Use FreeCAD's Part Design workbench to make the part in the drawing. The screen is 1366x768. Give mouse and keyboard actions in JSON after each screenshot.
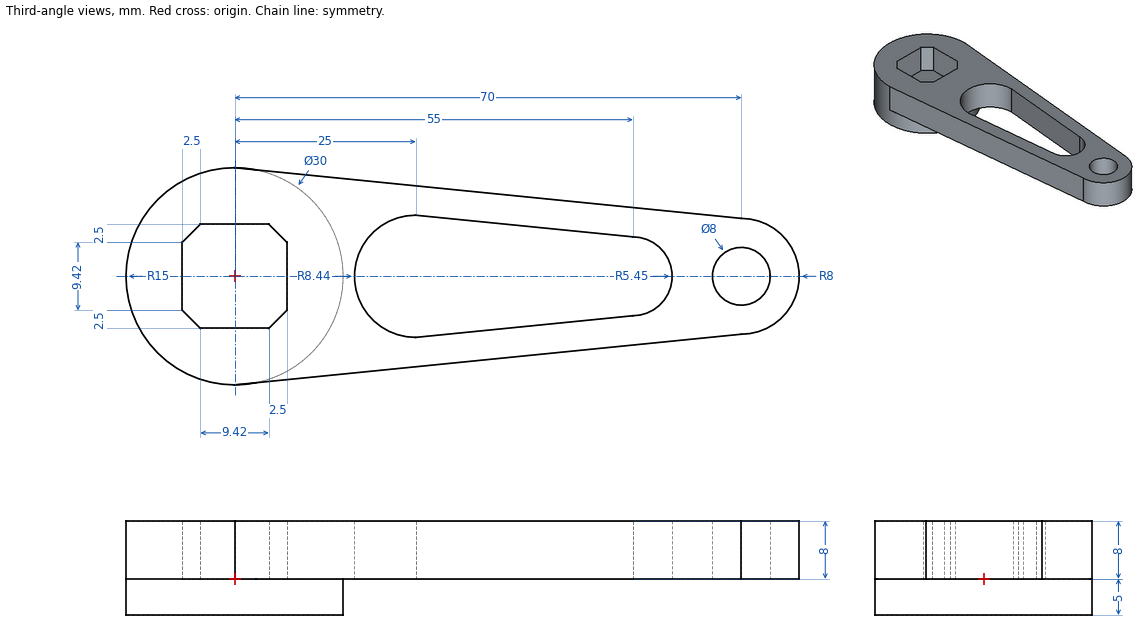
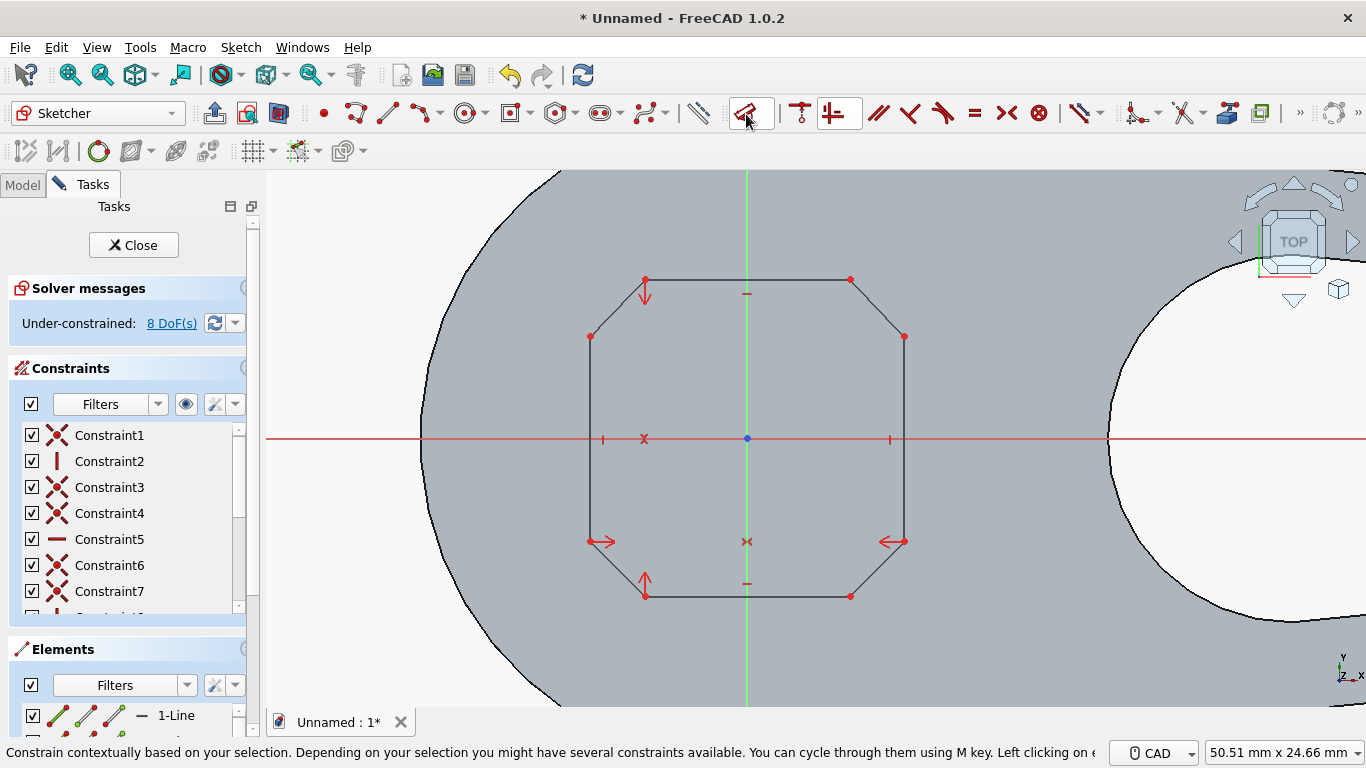
{"action": "left_click", "coordinate": [590, 398]}
{"action": "left_click", "coordinate": [556, 392]}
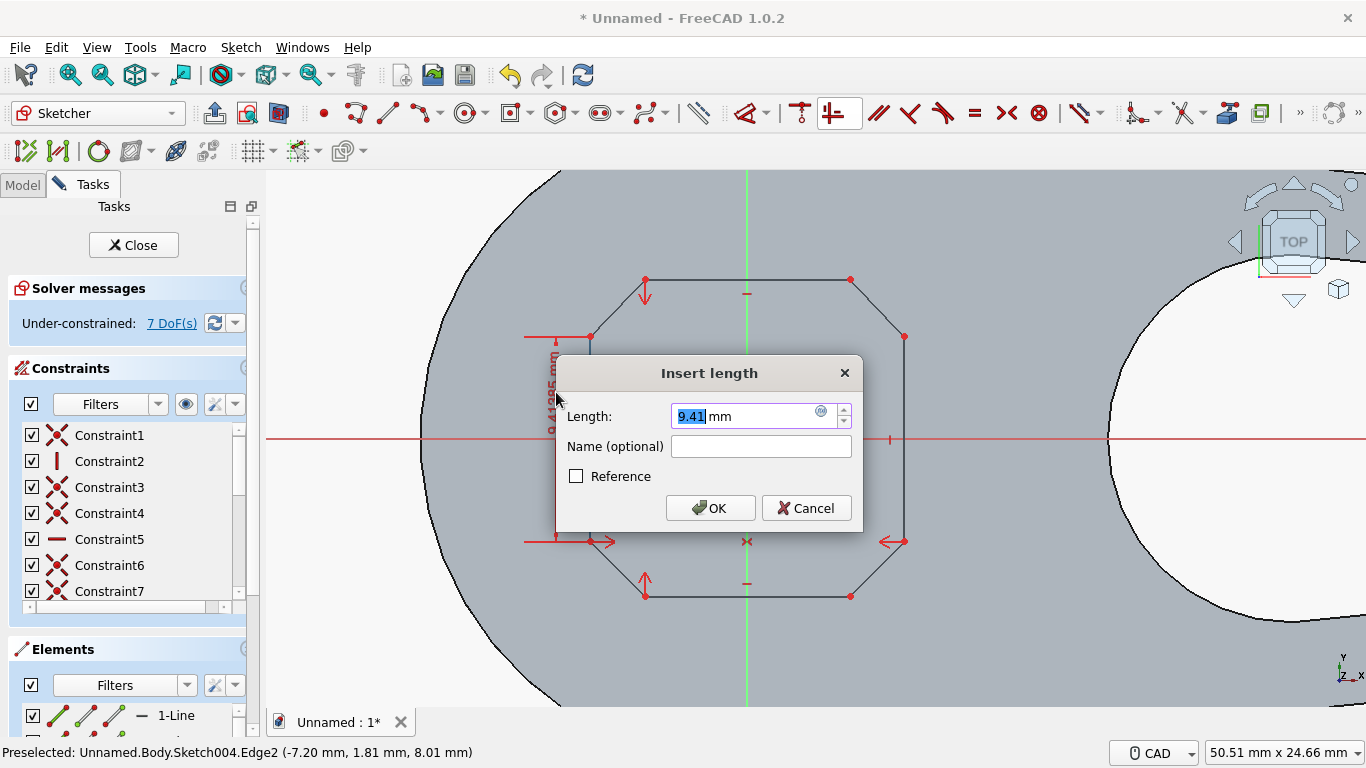
{"action": "type", "text": "9.42"}
{"action": "key", "text": "Return"}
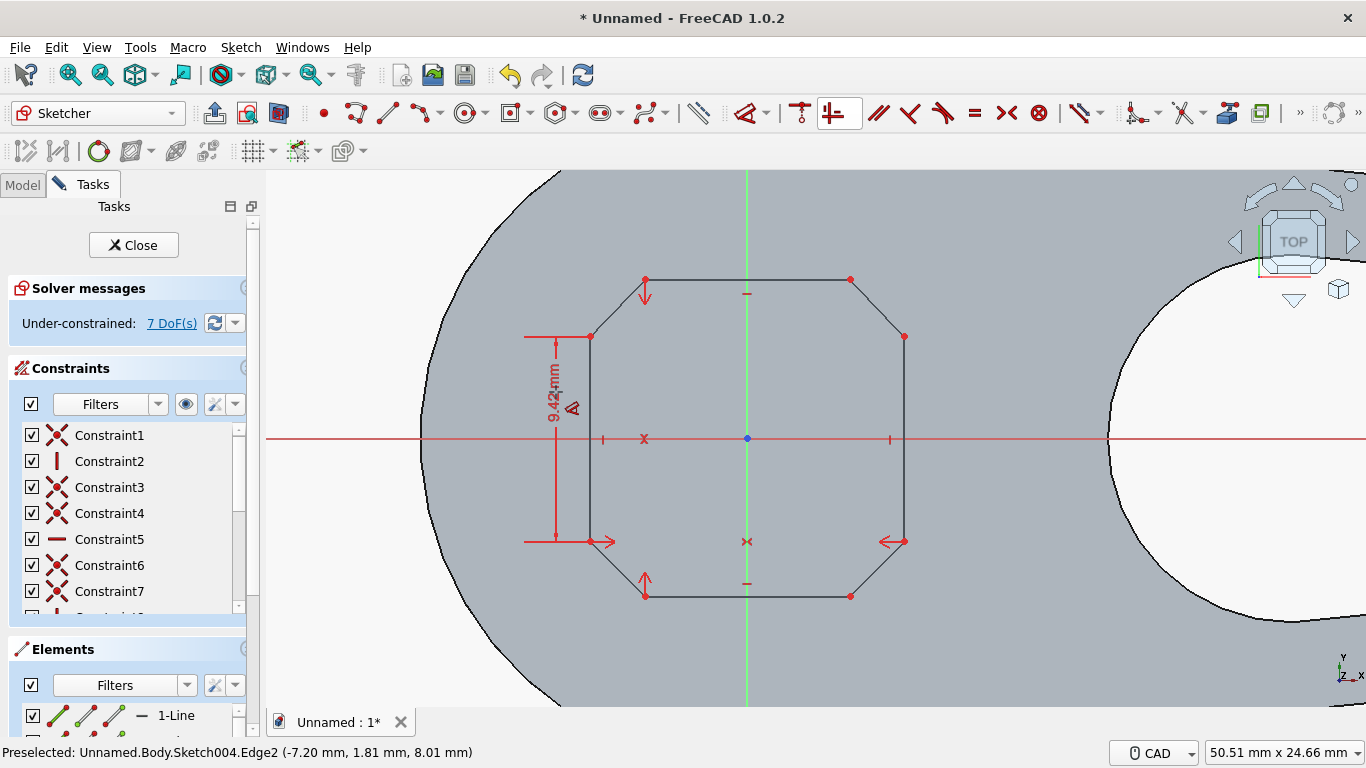
{"action": "left_click", "coordinate": [706, 597]}
{"action": "left_click", "coordinate": [700, 631]}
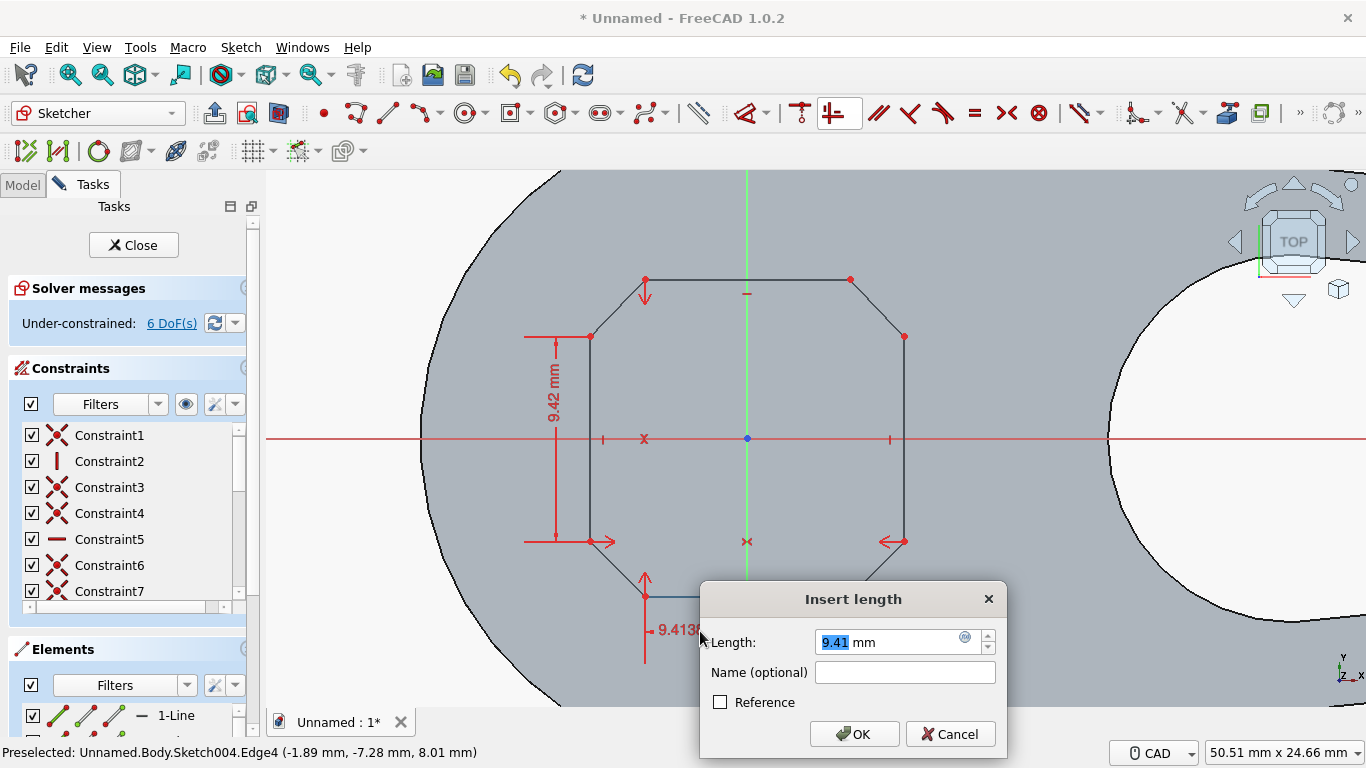
{"action": "type", "text": "9.42"}
{"action": "key", "text": "Return"}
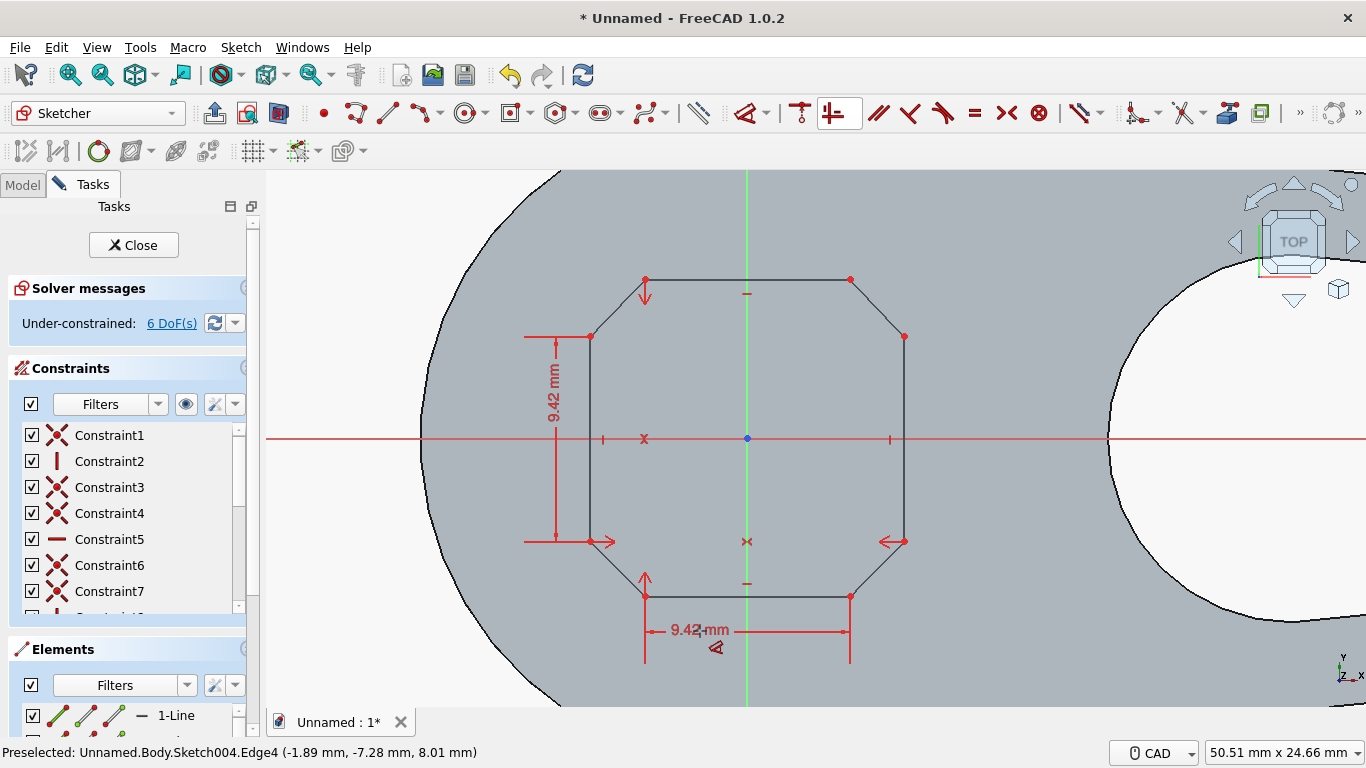
{"action": "left_click", "coordinate": [904, 480]}
{"action": "left_click", "coordinate": [938, 392]}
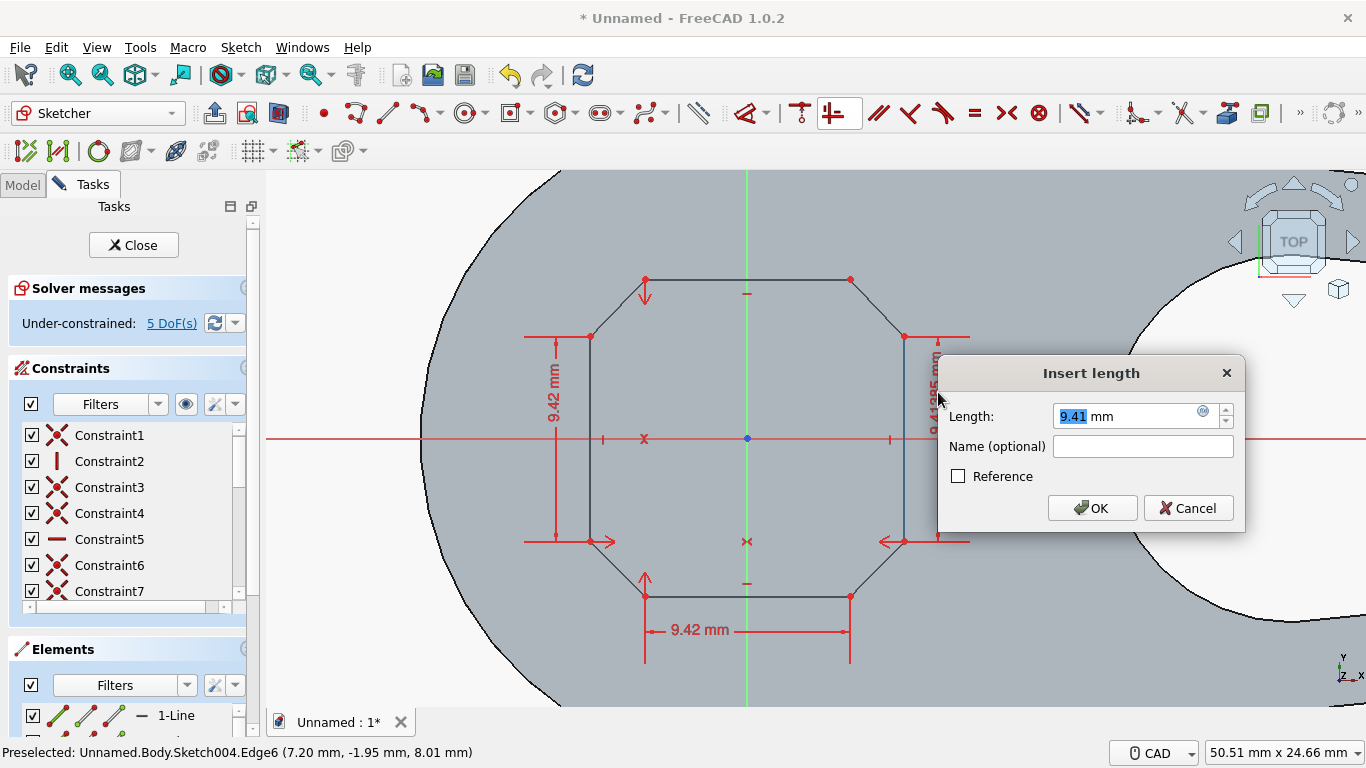
{"action": "type", "text": "9.42"}
{"action": "key", "text": "Return"}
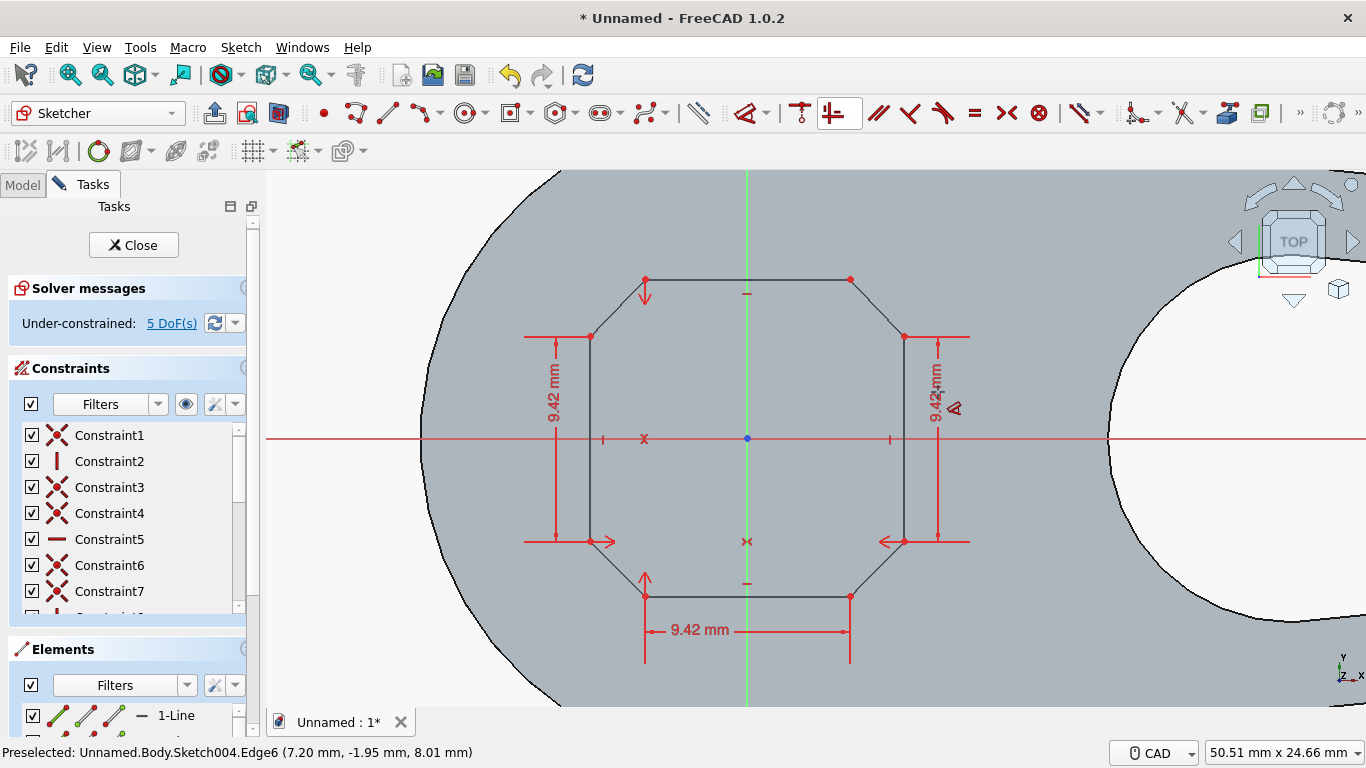
{"action": "left_click", "coordinate": [788, 280]}
{"action": "left_click", "coordinate": [700, 246]}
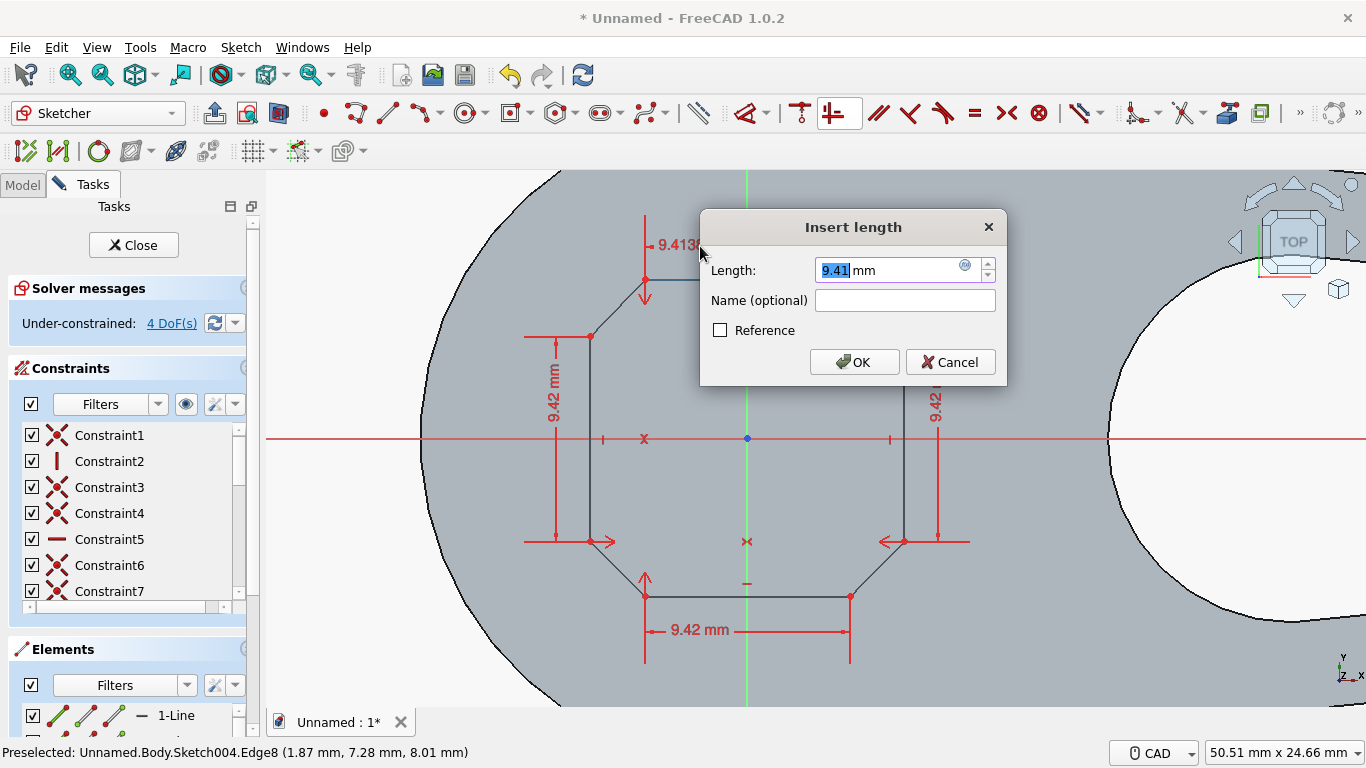
{"action": "type", "text": "9.42"}
{"action": "key", "text": "Return"}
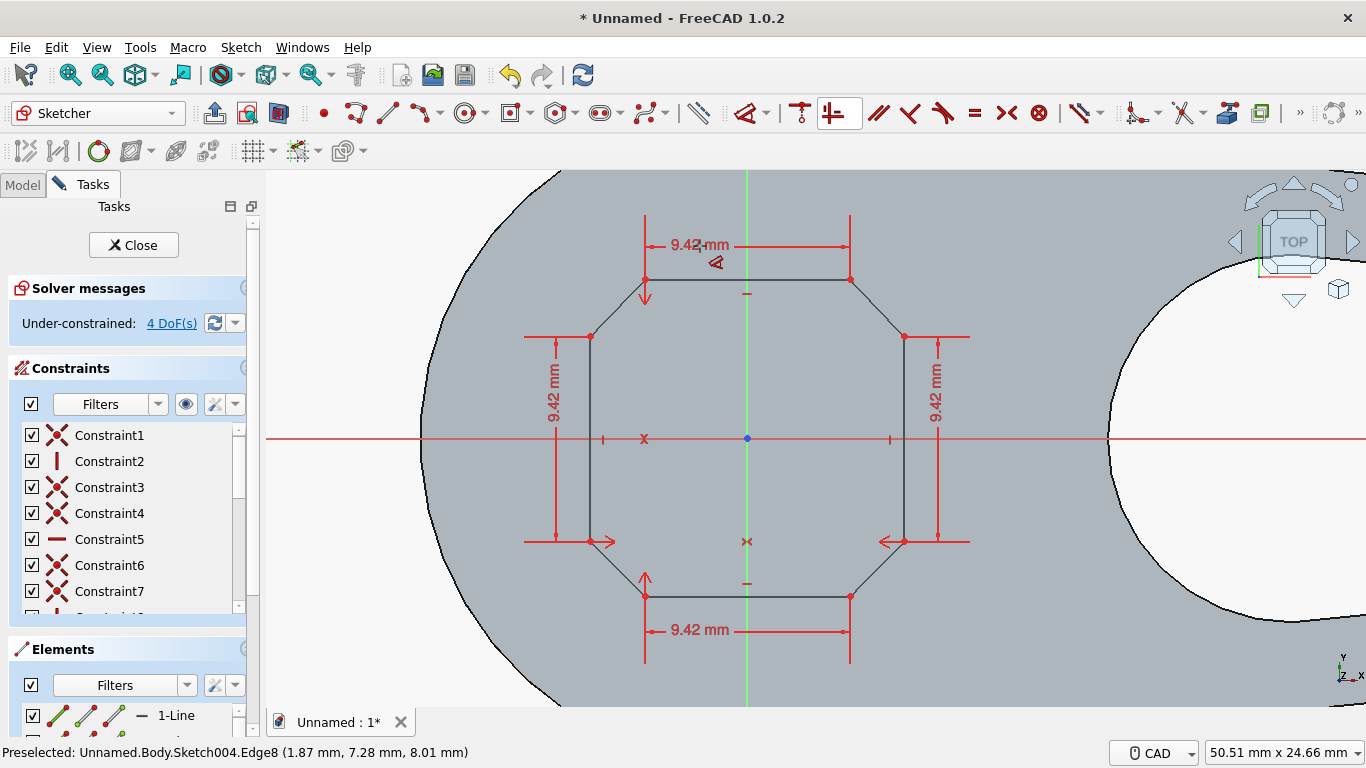
{"action": "left_click", "coordinate": [629, 297]}
{"action": "left_click", "coordinate": [618, 246]}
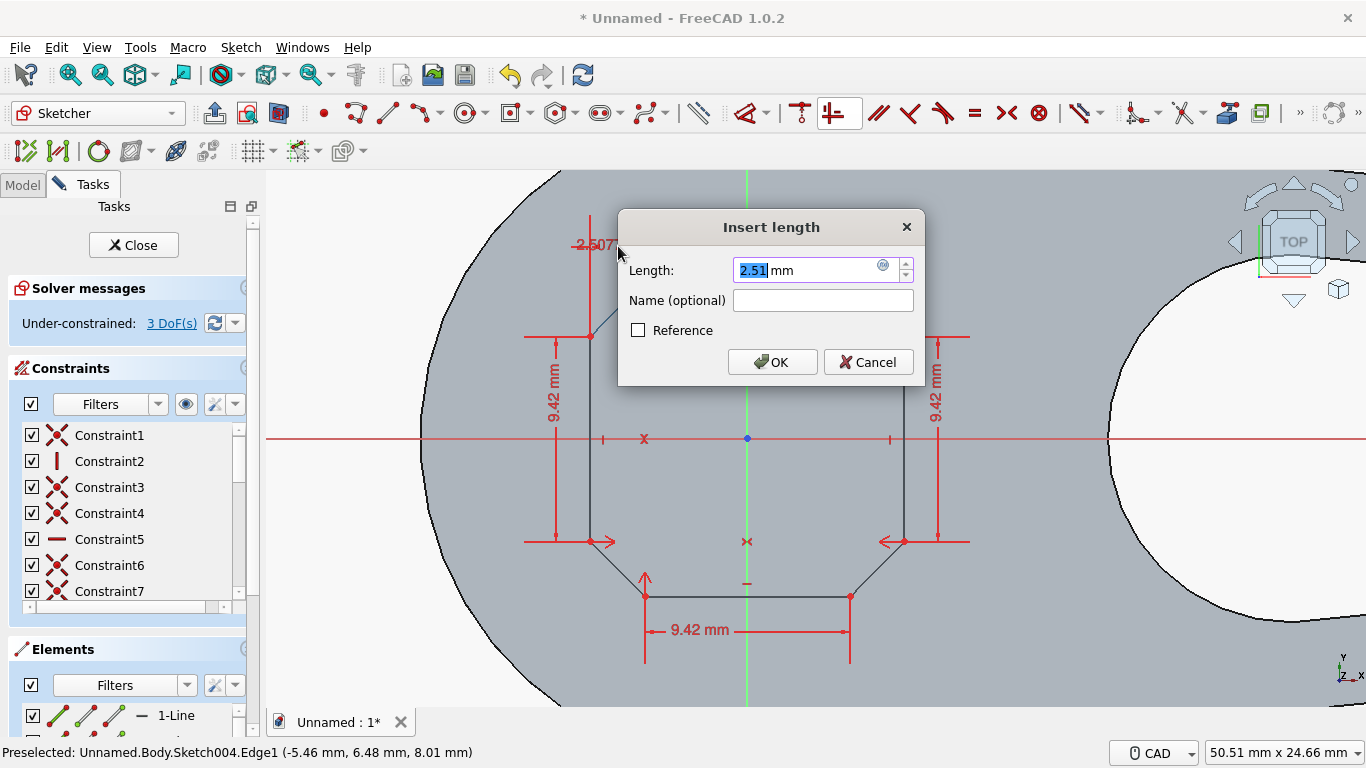
{"action": "type", "text": "2.5"}
{"action": "key", "text": "Return"}